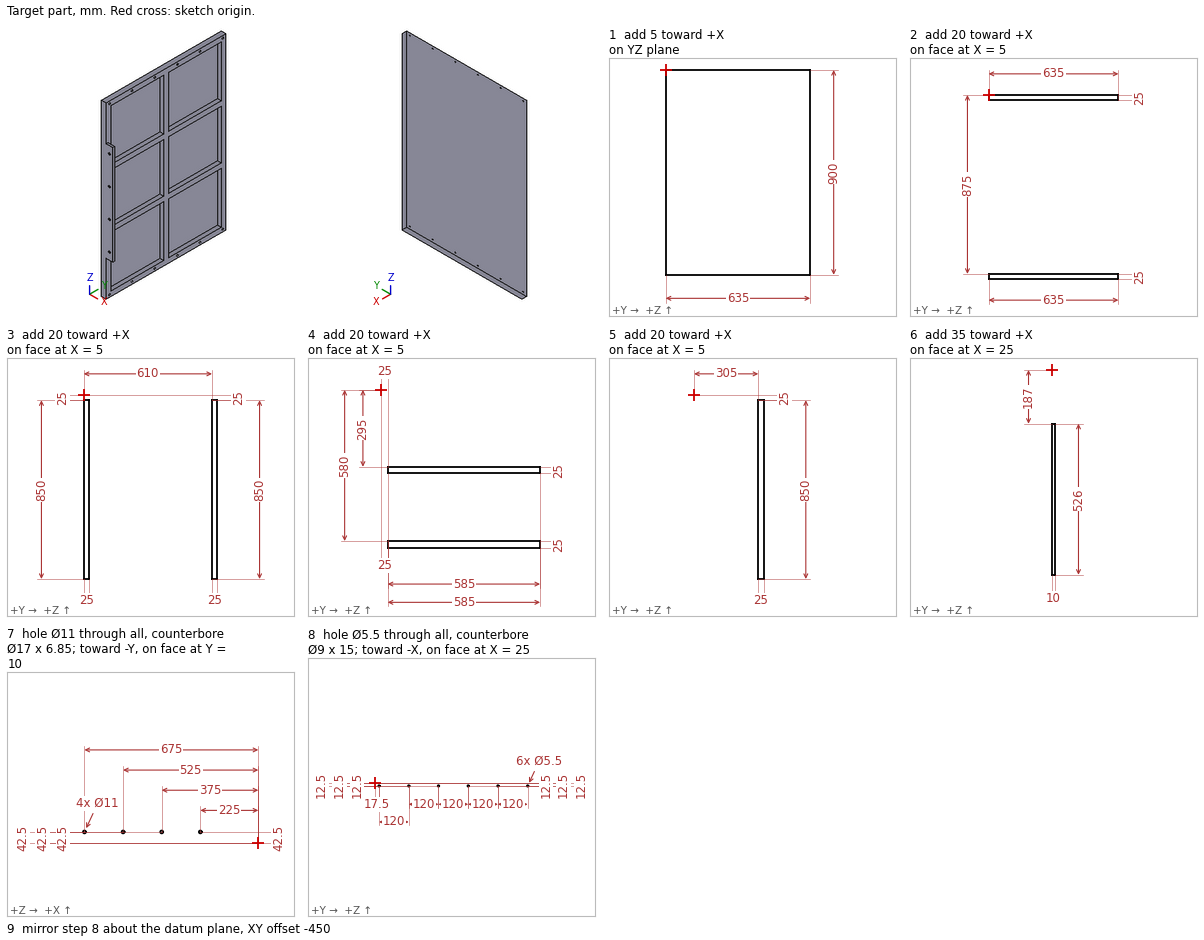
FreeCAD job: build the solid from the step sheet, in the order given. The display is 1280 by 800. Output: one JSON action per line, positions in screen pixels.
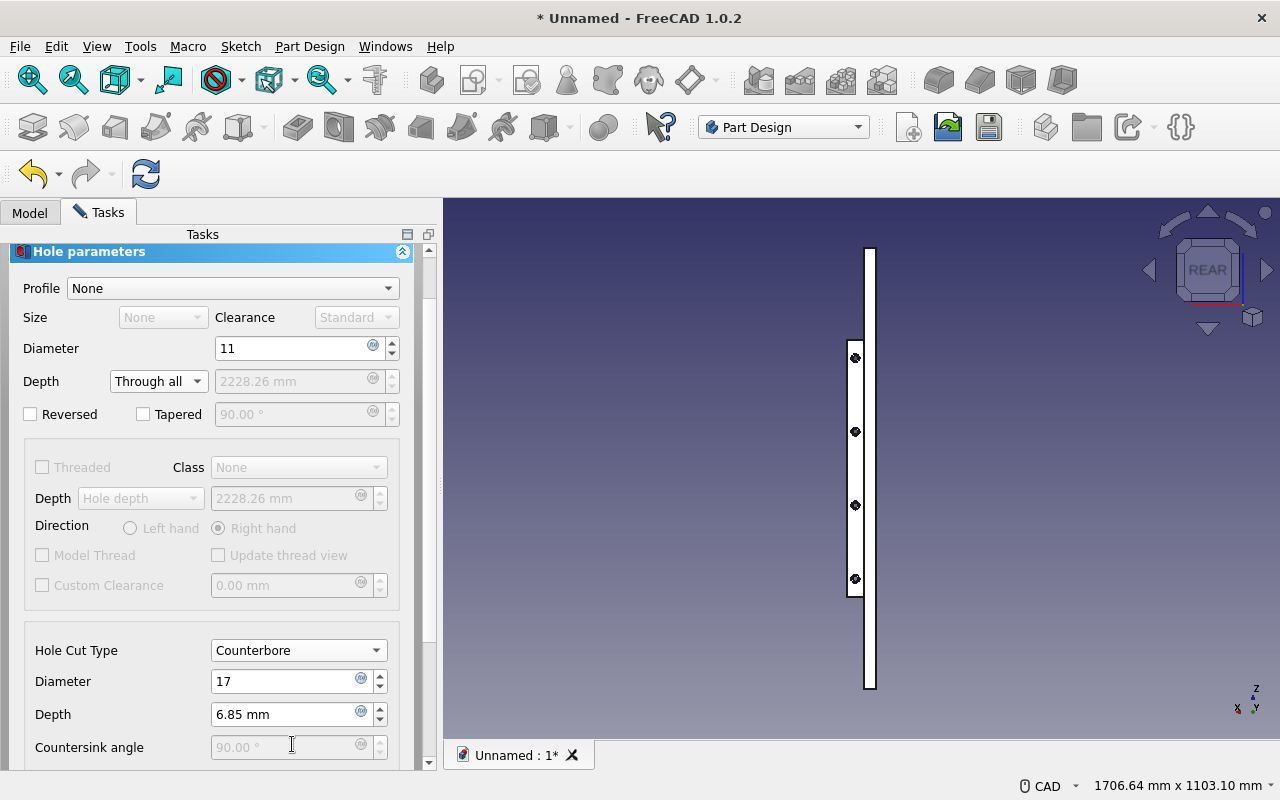
{"action": "scroll", "coordinate": [429, 507], "scroll_direction": "up", "scroll_amount": 2}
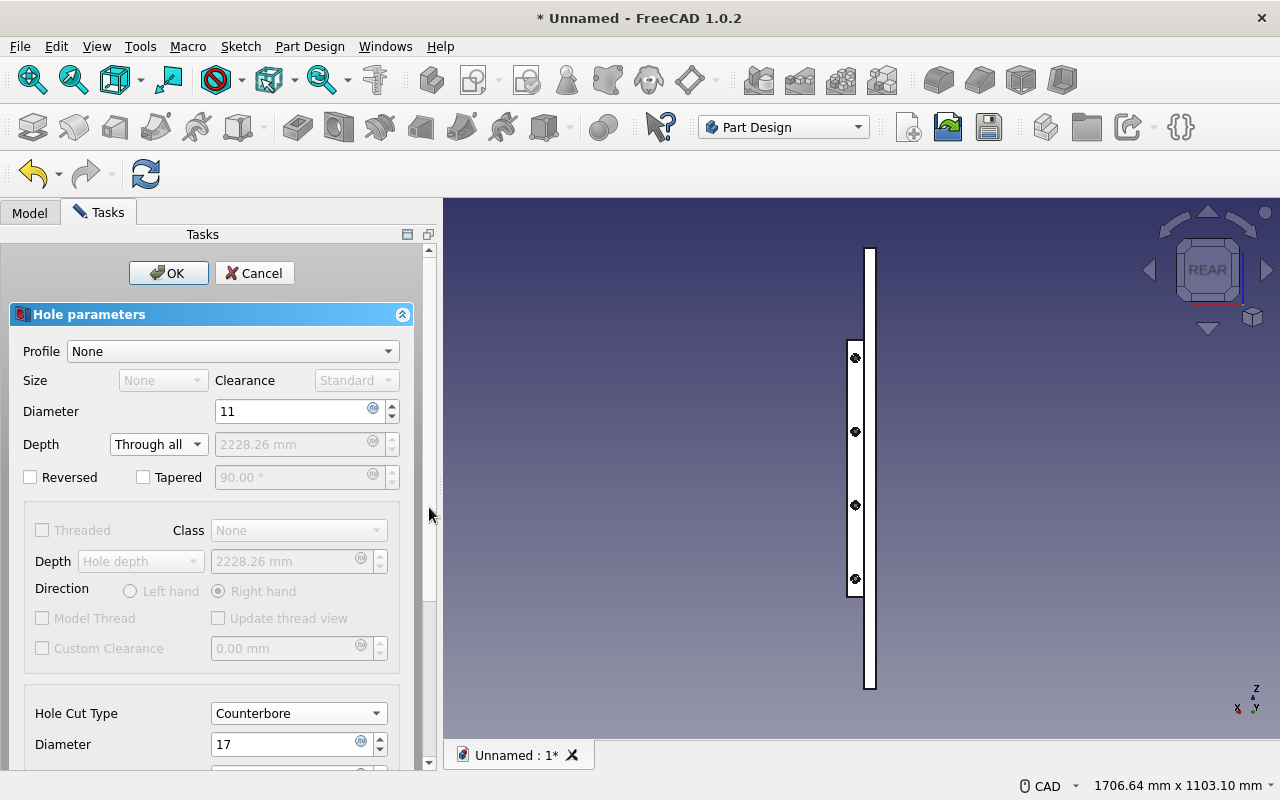
{"action": "left_click", "coordinate": [169, 273]}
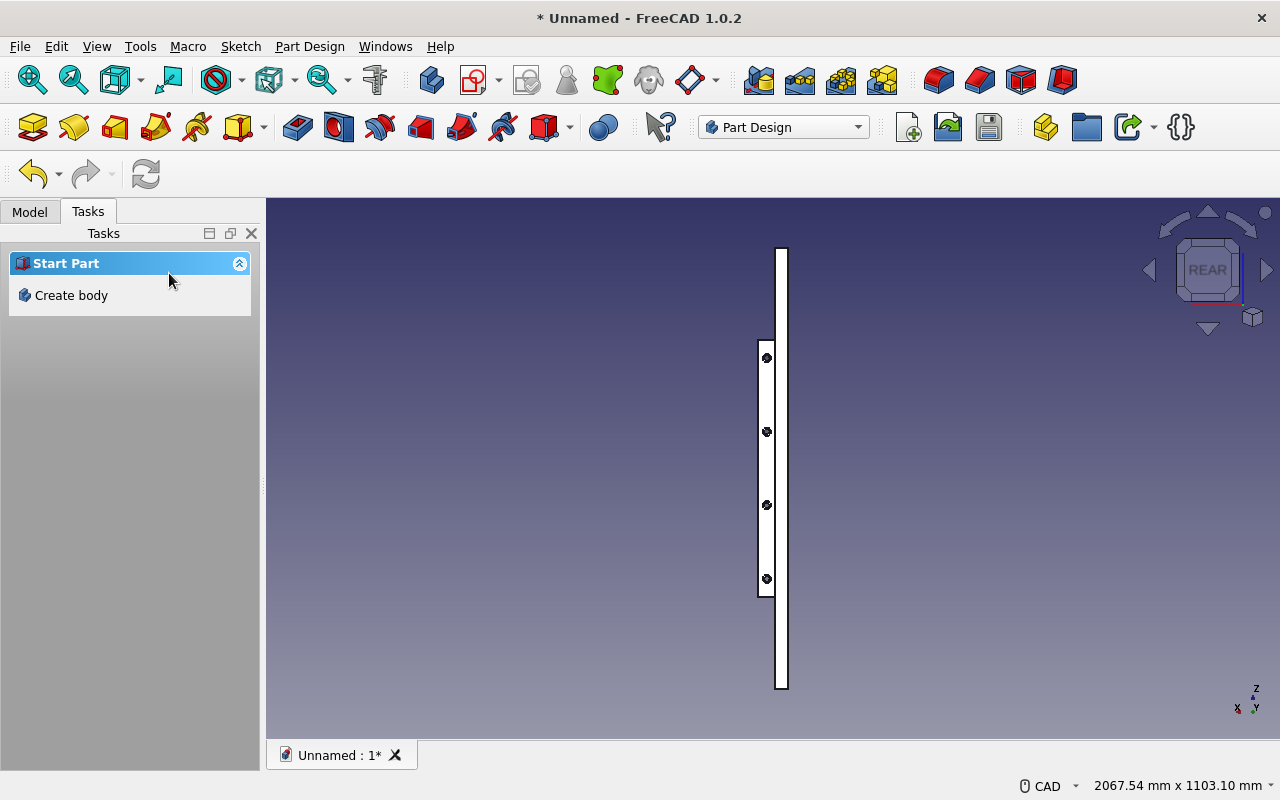
{"action": "key", "text": "0"}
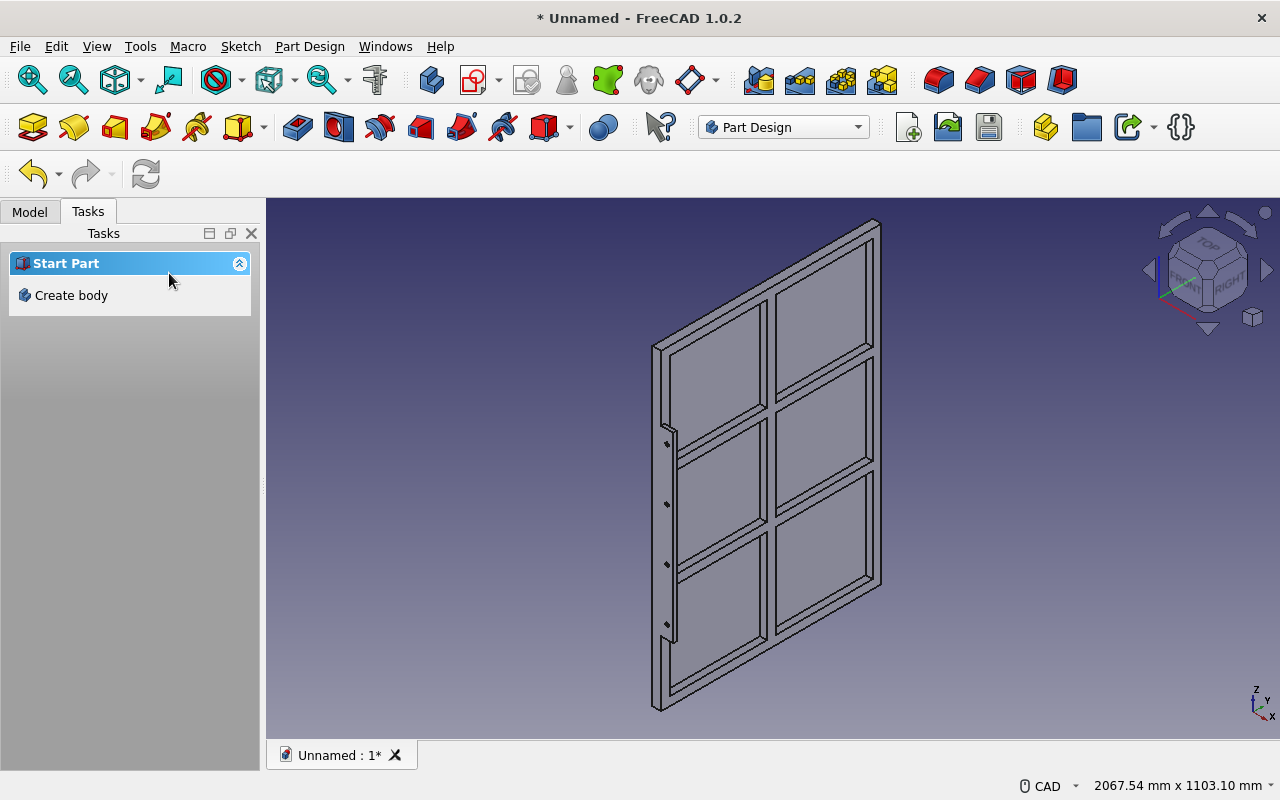
{"action": "scroll", "coordinate": [771, 621], "scroll_direction": "up", "scroll_amount": 4}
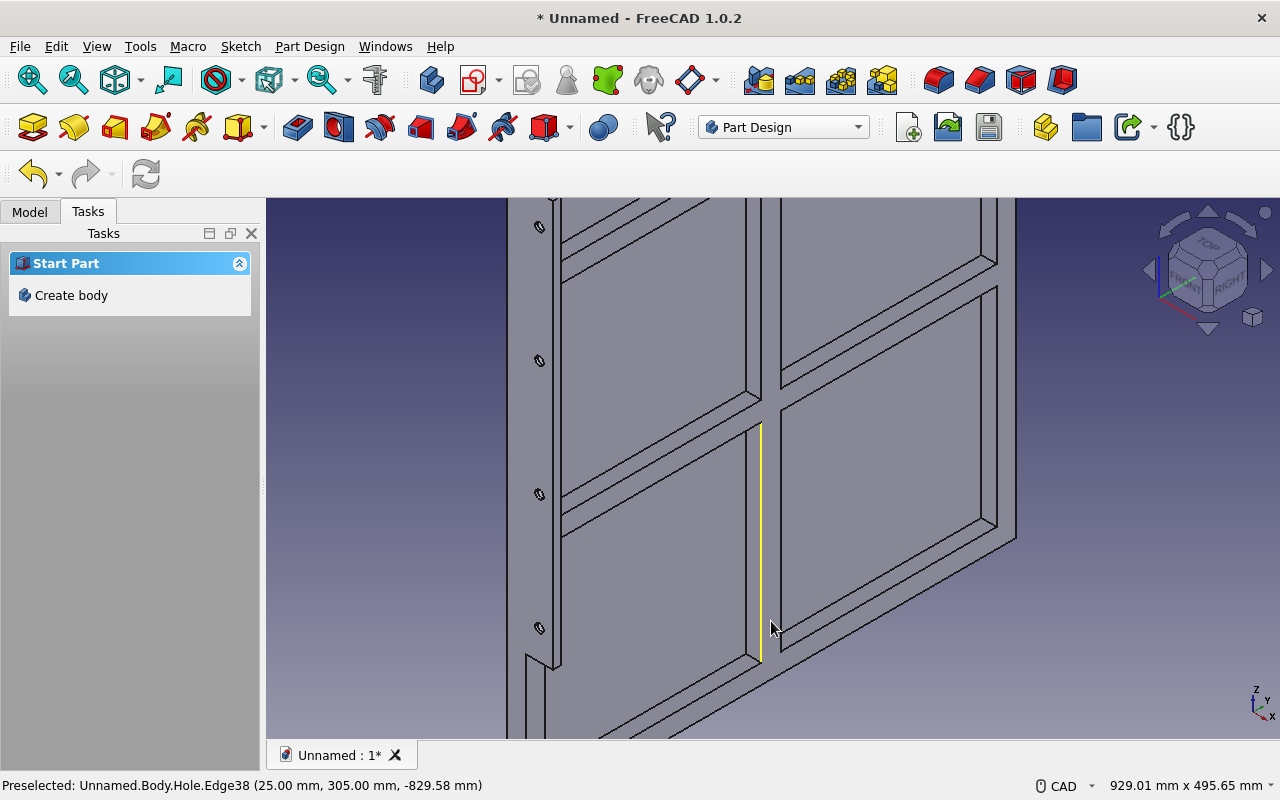
{"action": "left_click", "coordinate": [771, 621]}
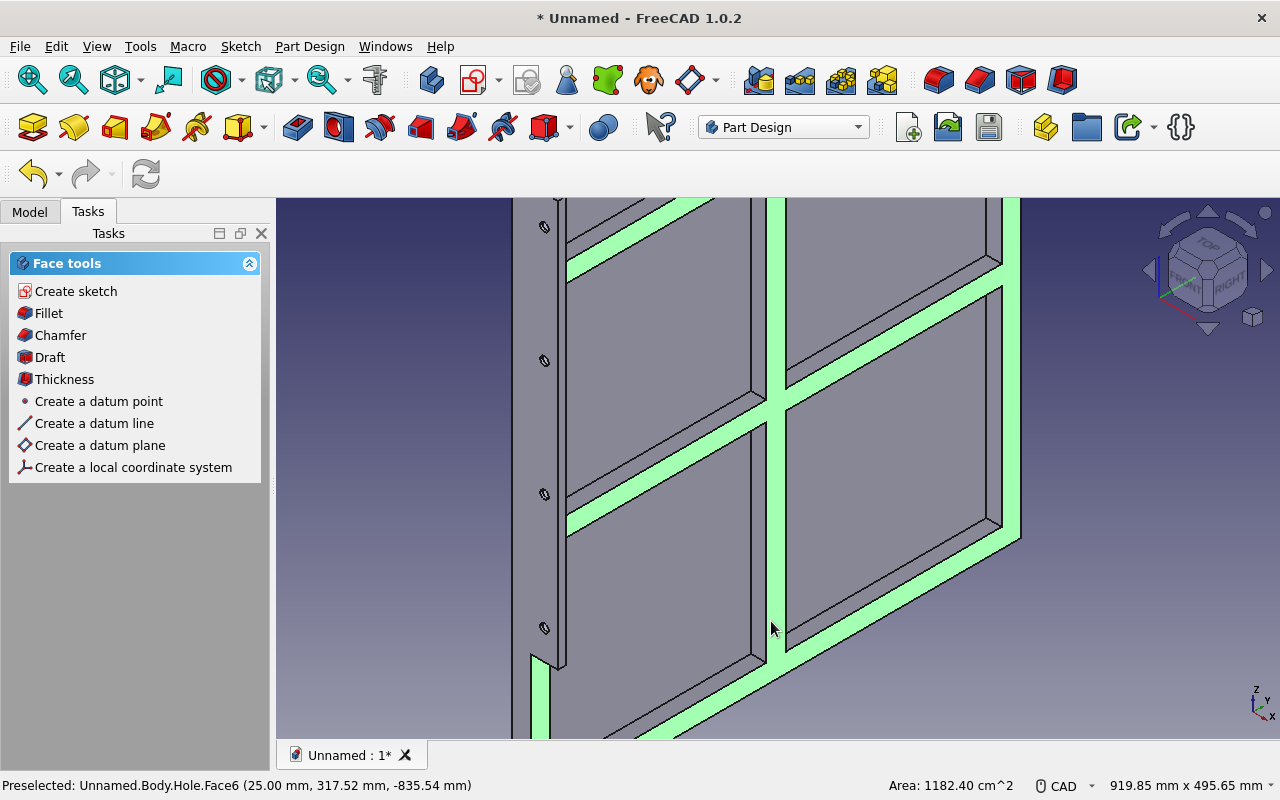
{"action": "left_click", "coordinate": [472, 80]}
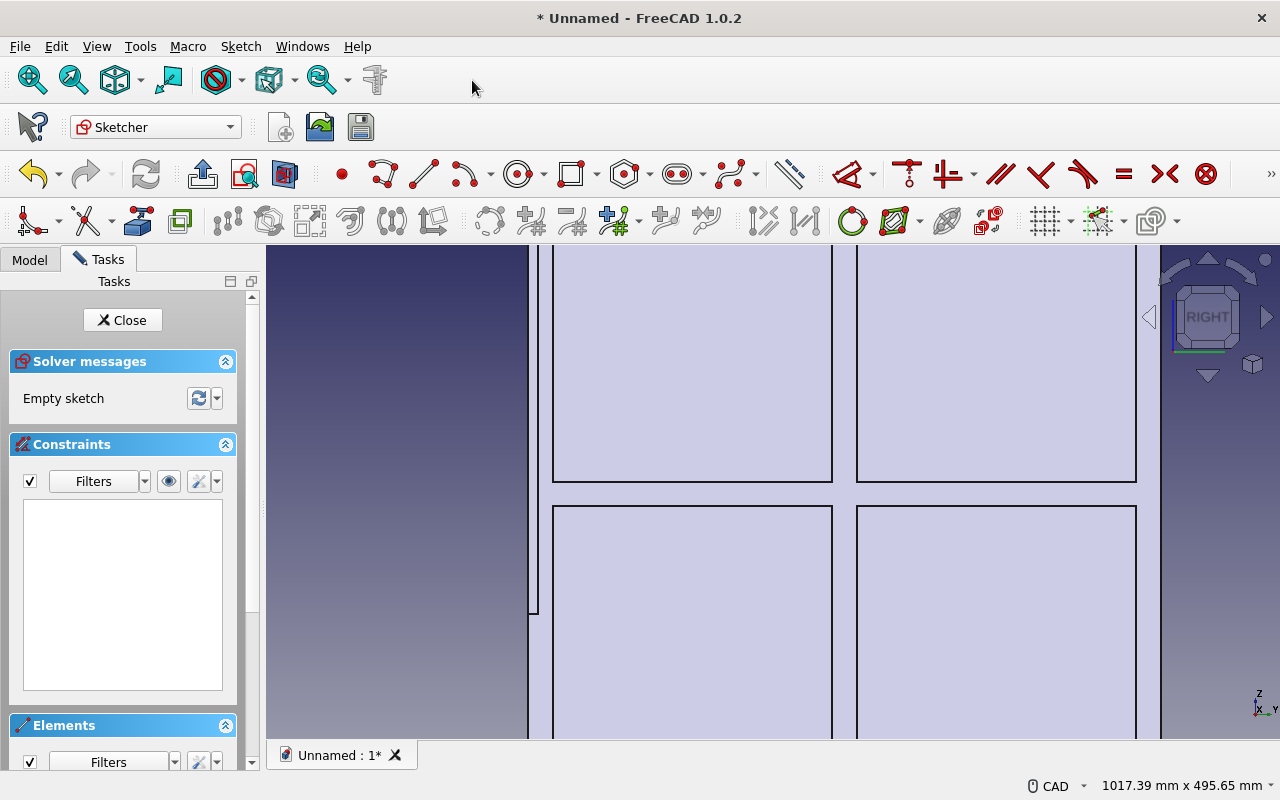
{"action": "left_click", "coordinate": [285, 174]}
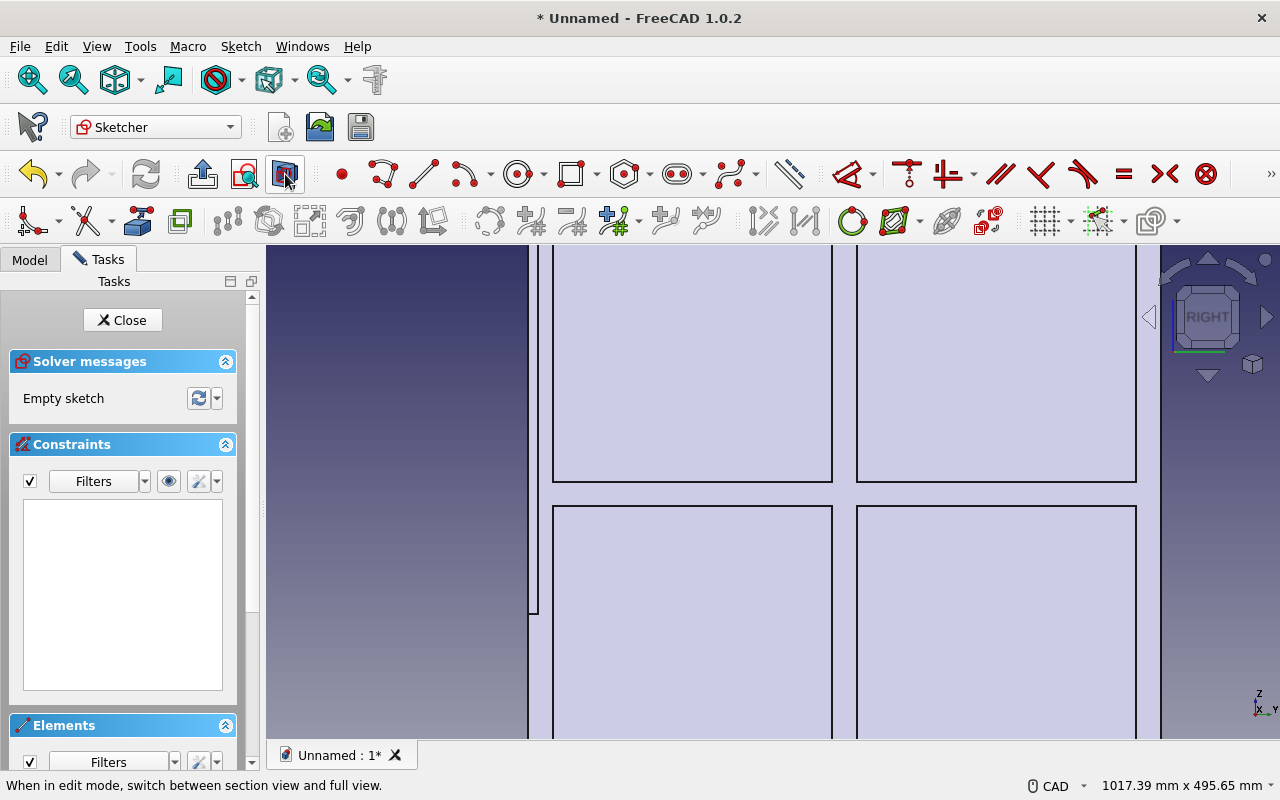
{"action": "scroll", "coordinate": [704, 492], "scroll_direction": "down", "scroll_amount": 5}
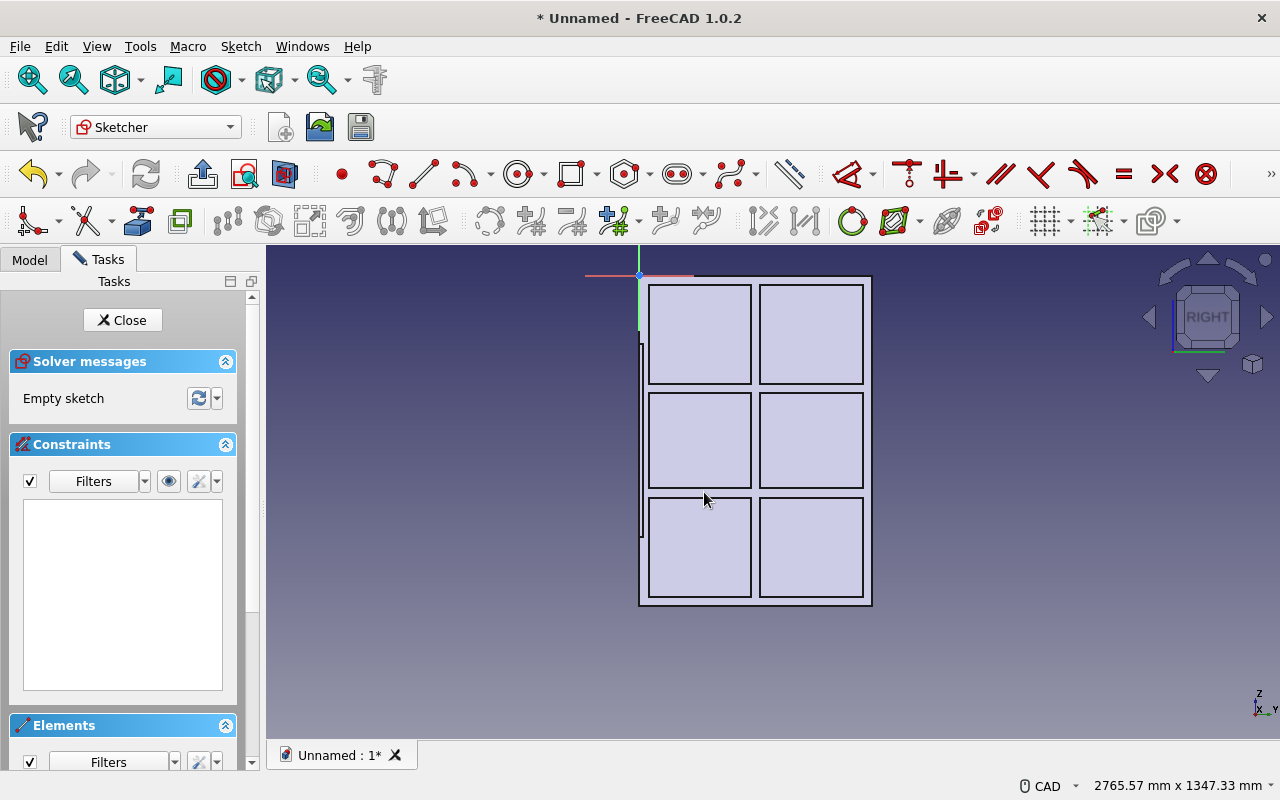
{"action": "scroll", "coordinate": [704, 492], "scroll_direction": "down", "scroll_amount": 5}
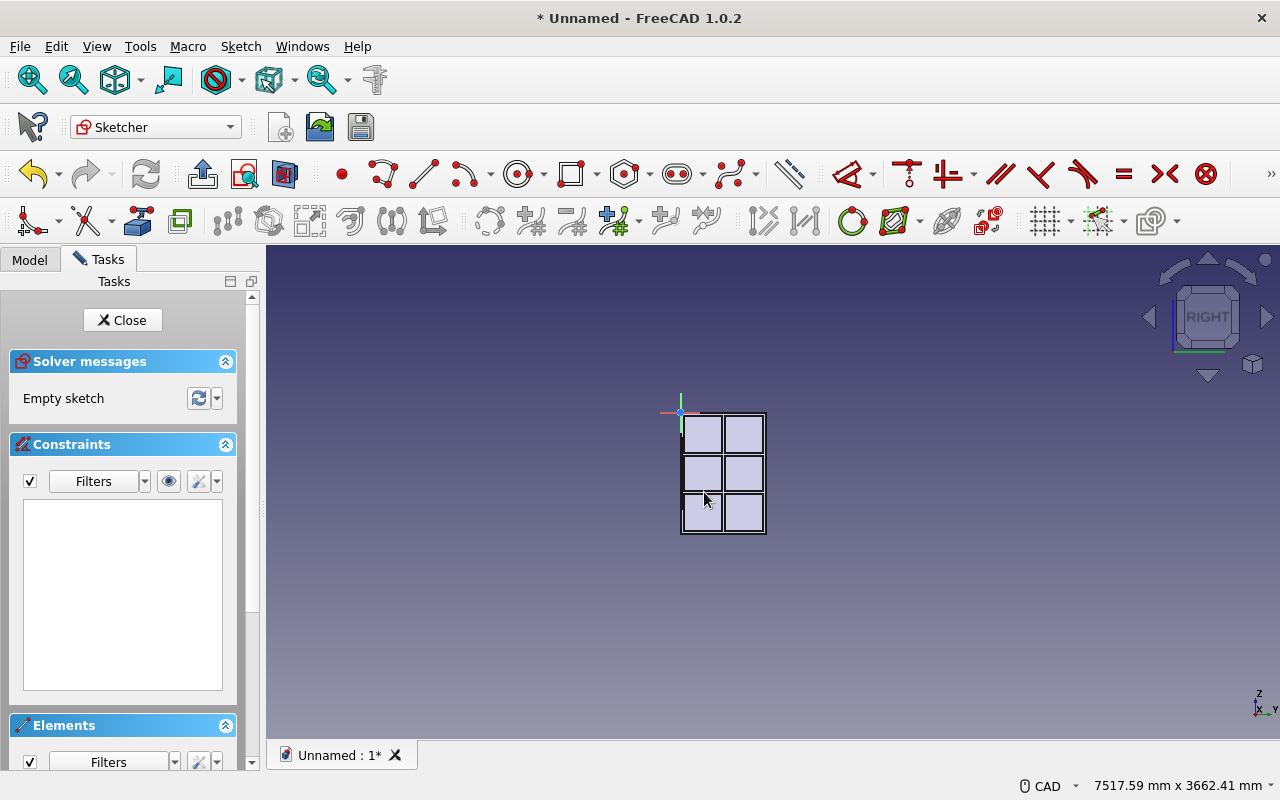
{"action": "scroll", "coordinate": [725, 402], "scroll_direction": "up", "scroll_amount": 10}